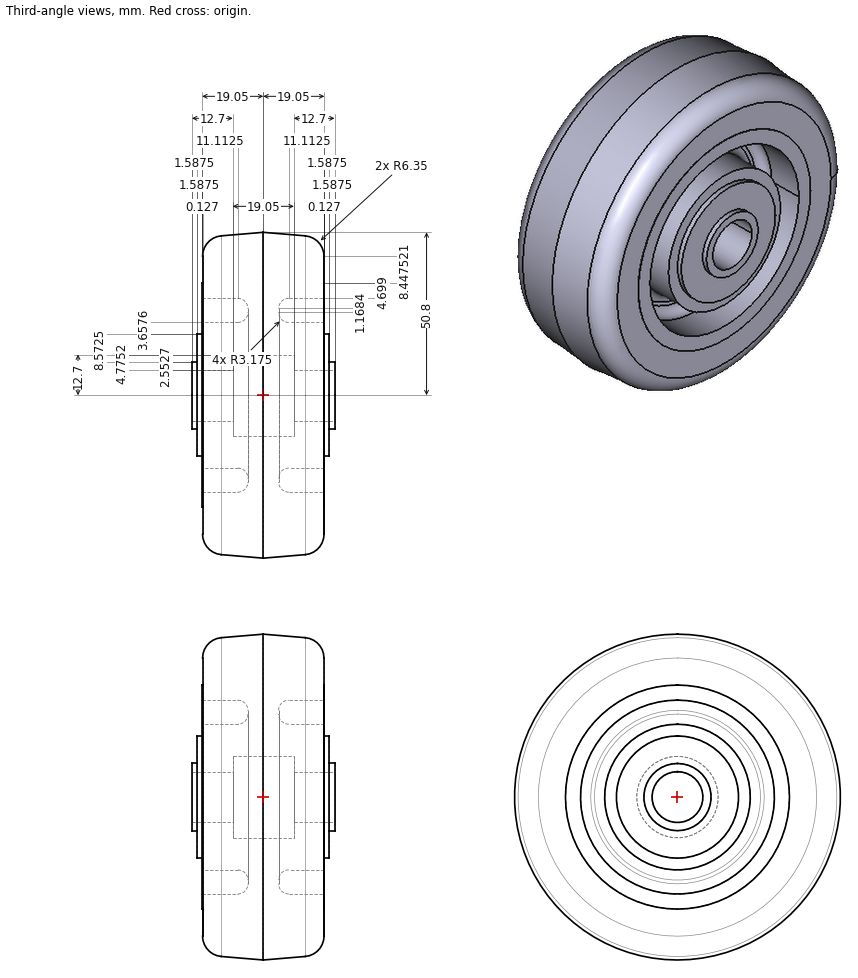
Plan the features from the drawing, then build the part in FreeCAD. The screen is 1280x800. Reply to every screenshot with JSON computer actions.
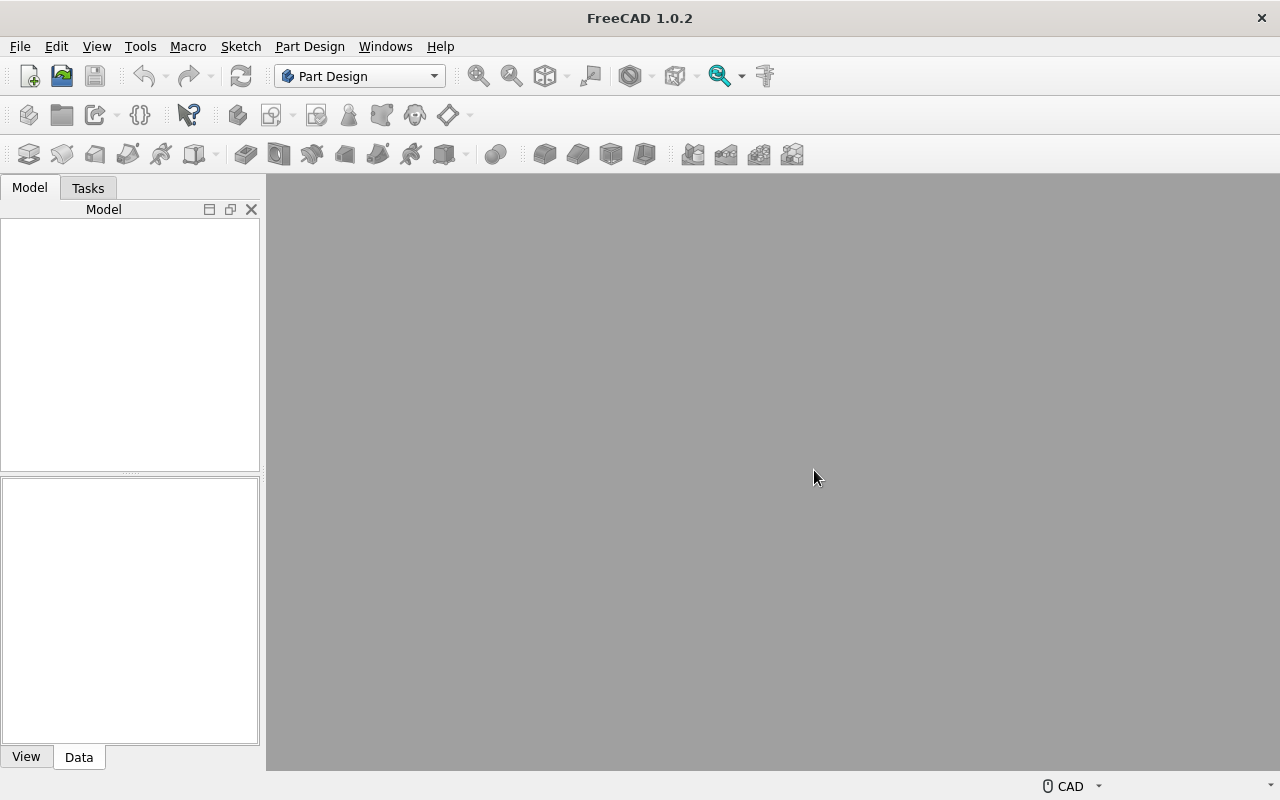
{"action": "left_click", "coordinate": [29, 76]}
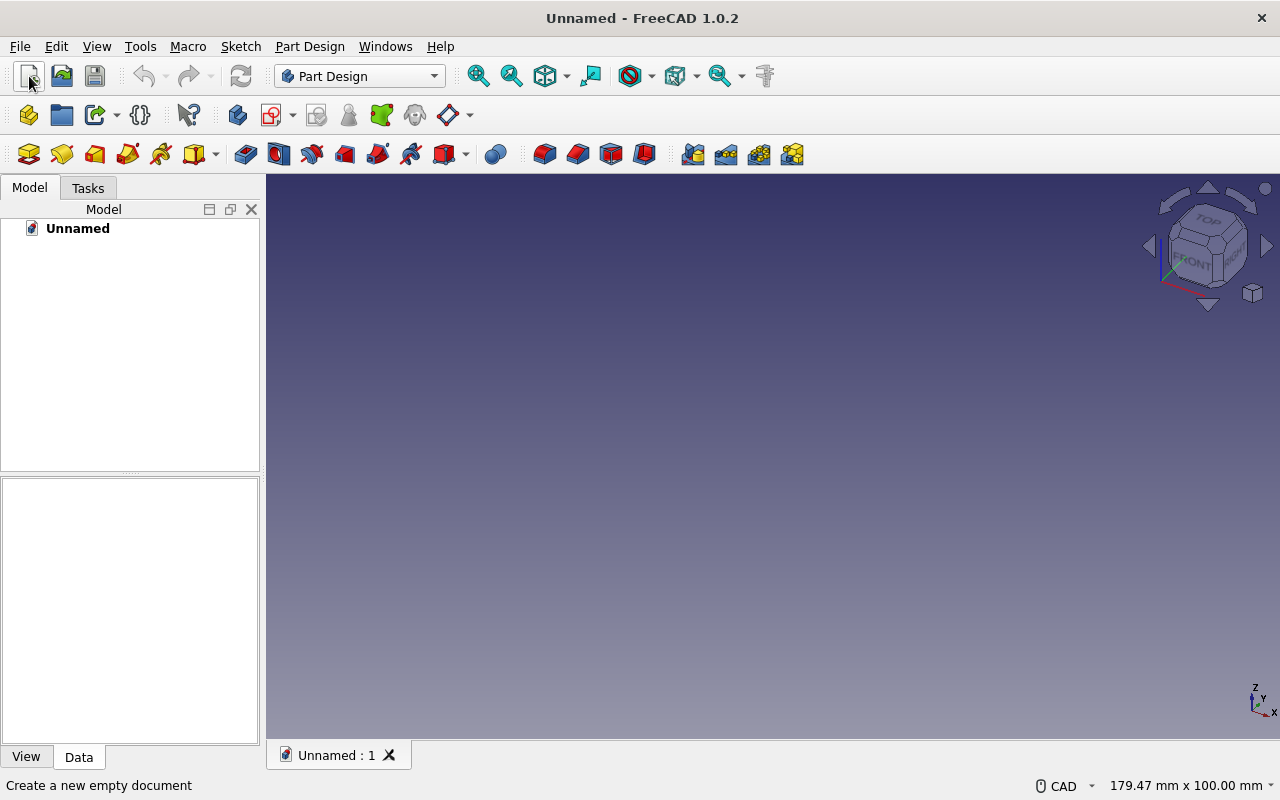
{"action": "left_click", "coordinate": [270, 116]}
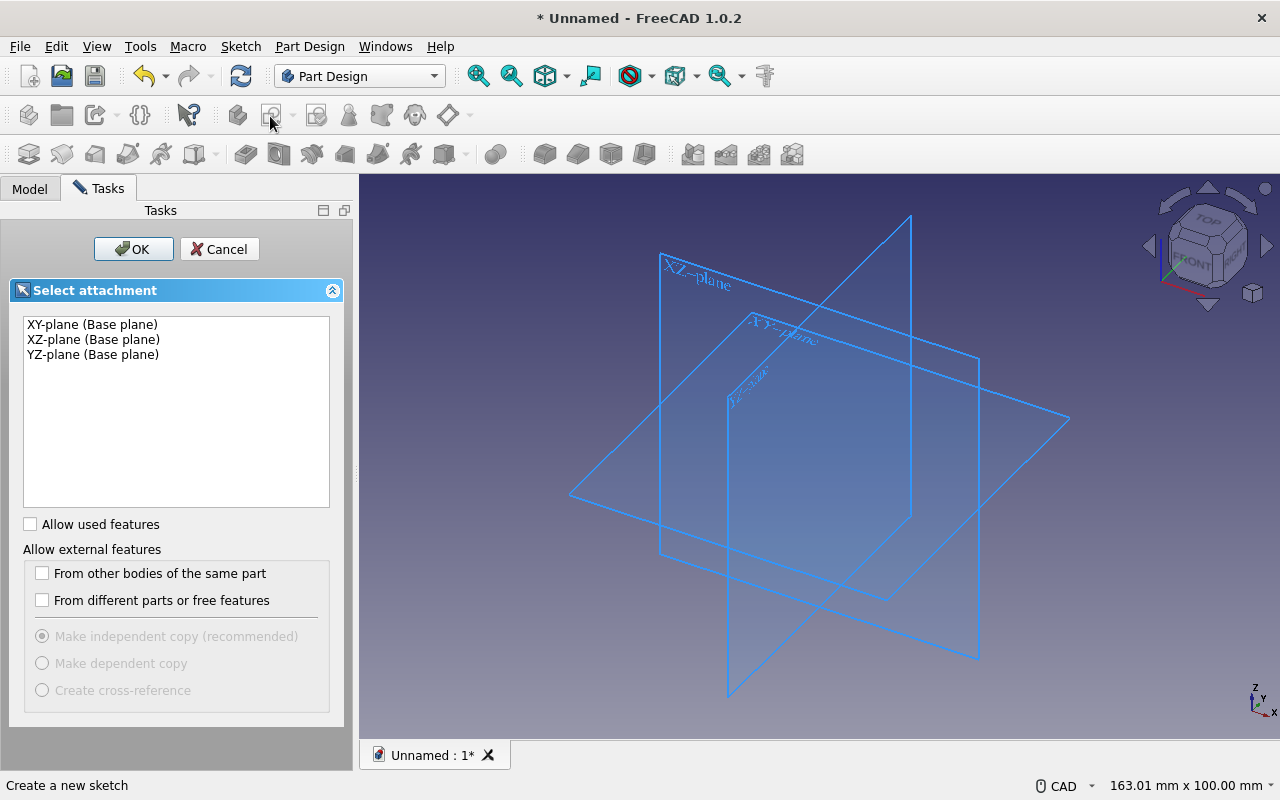
{"action": "left_click", "coordinate": [84, 324]}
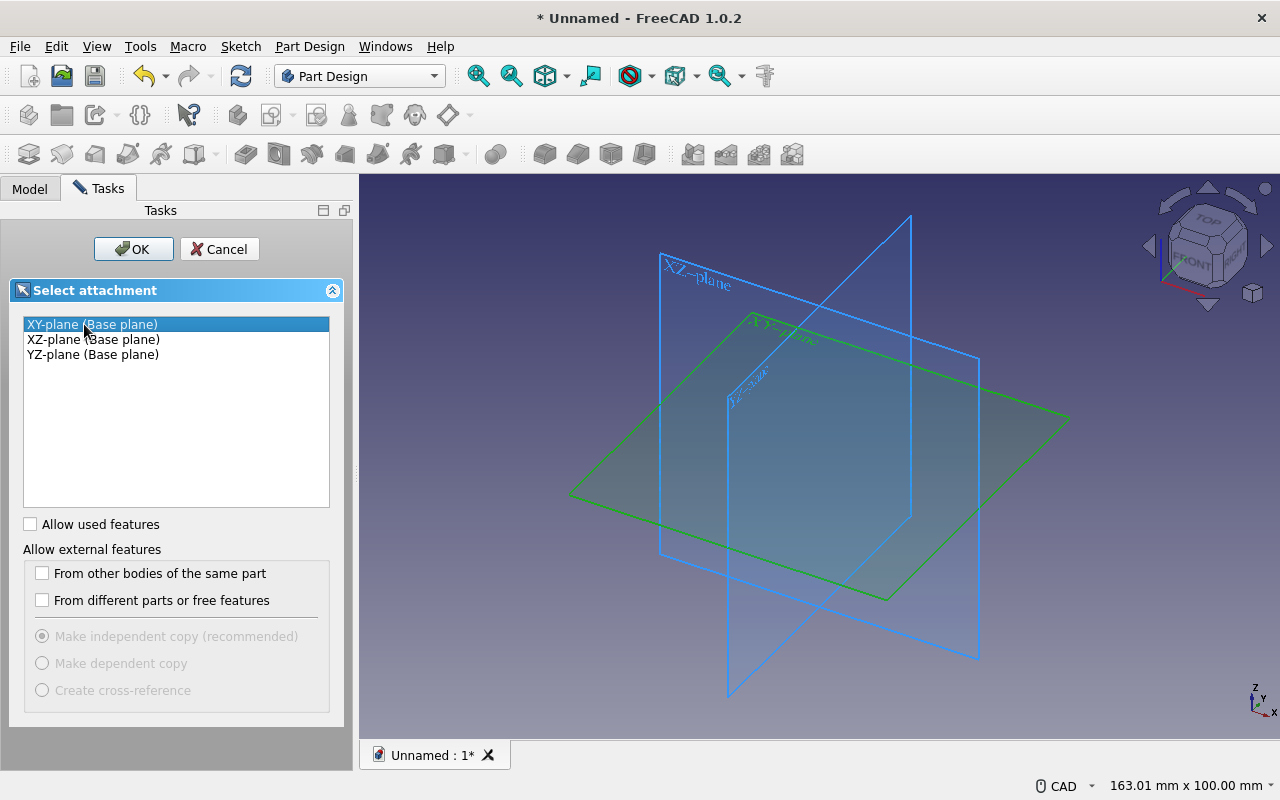
{"action": "left_click", "coordinate": [134, 249]}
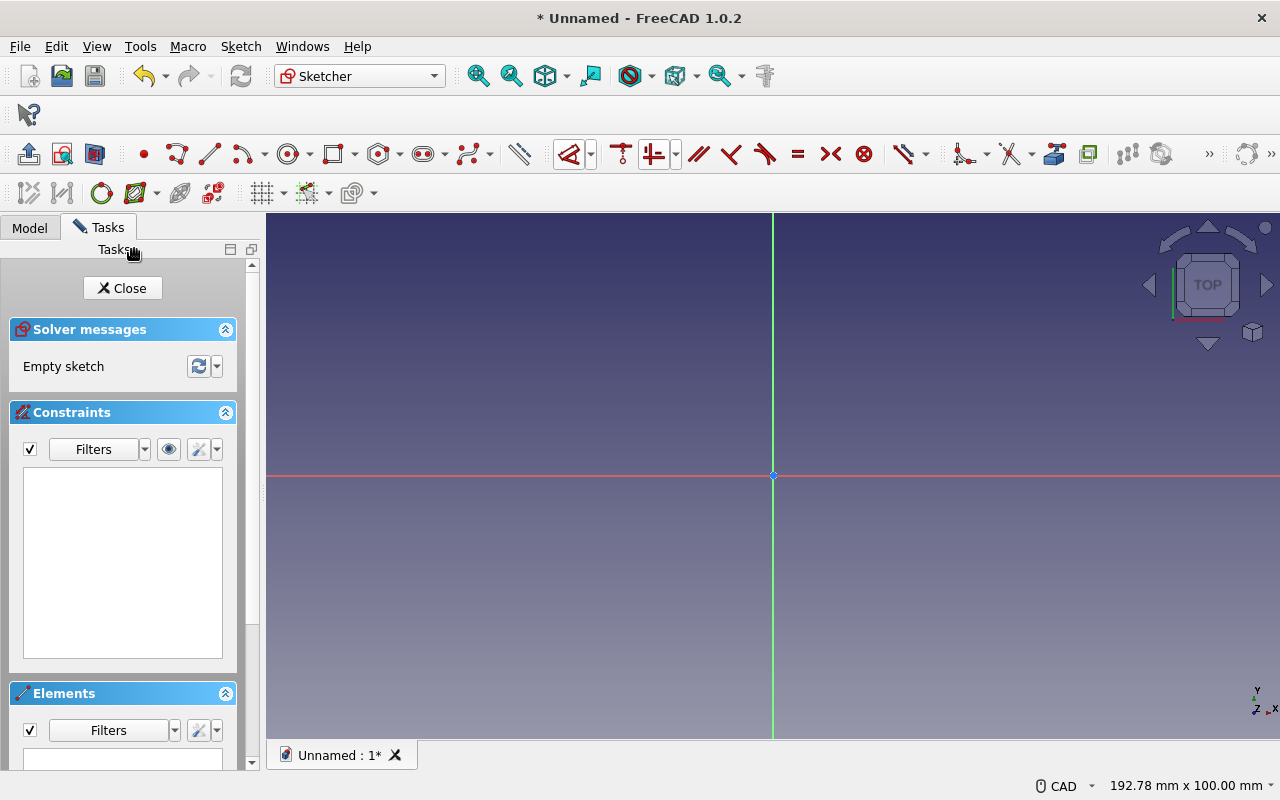
{"action": "scroll", "coordinate": [395, 711], "scroll_direction": "down", "scroll_amount": 1}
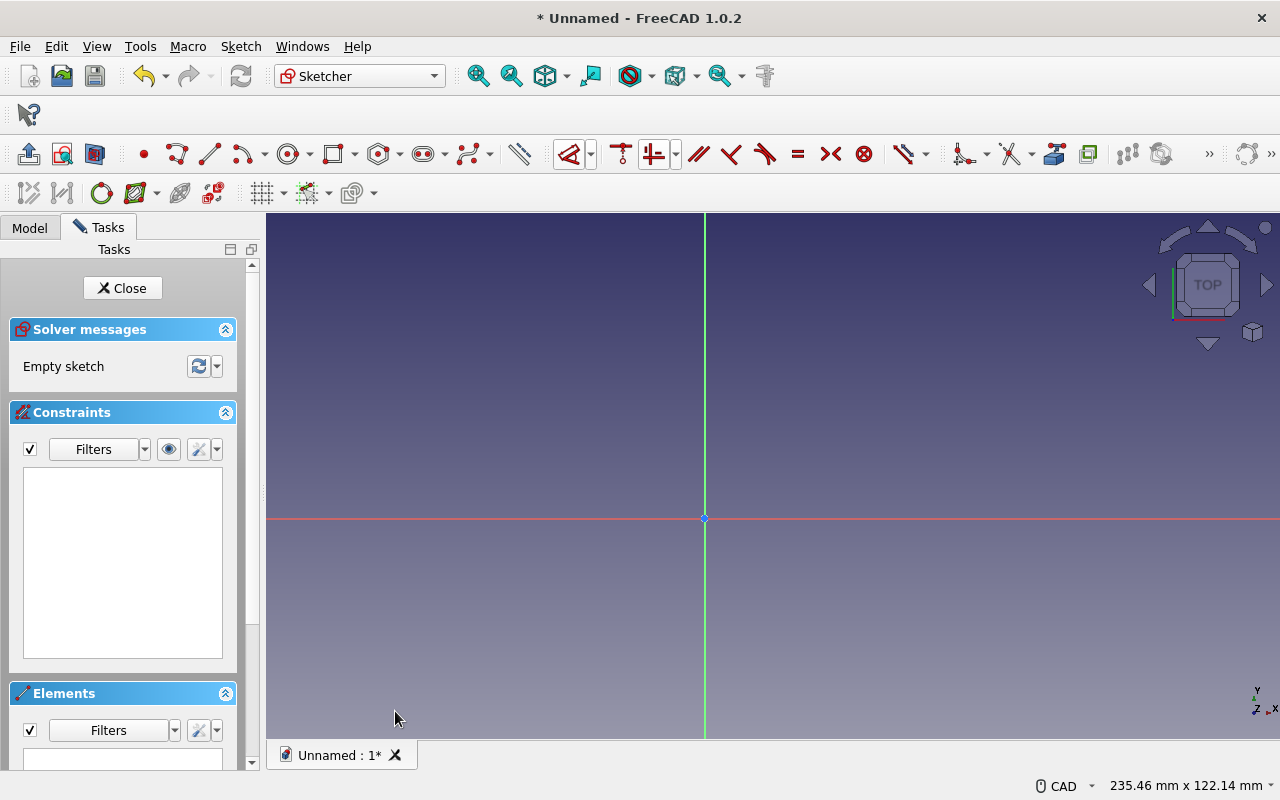
{"action": "scroll", "coordinate": [705, 274], "scroll_direction": "up", "scroll_amount": 2}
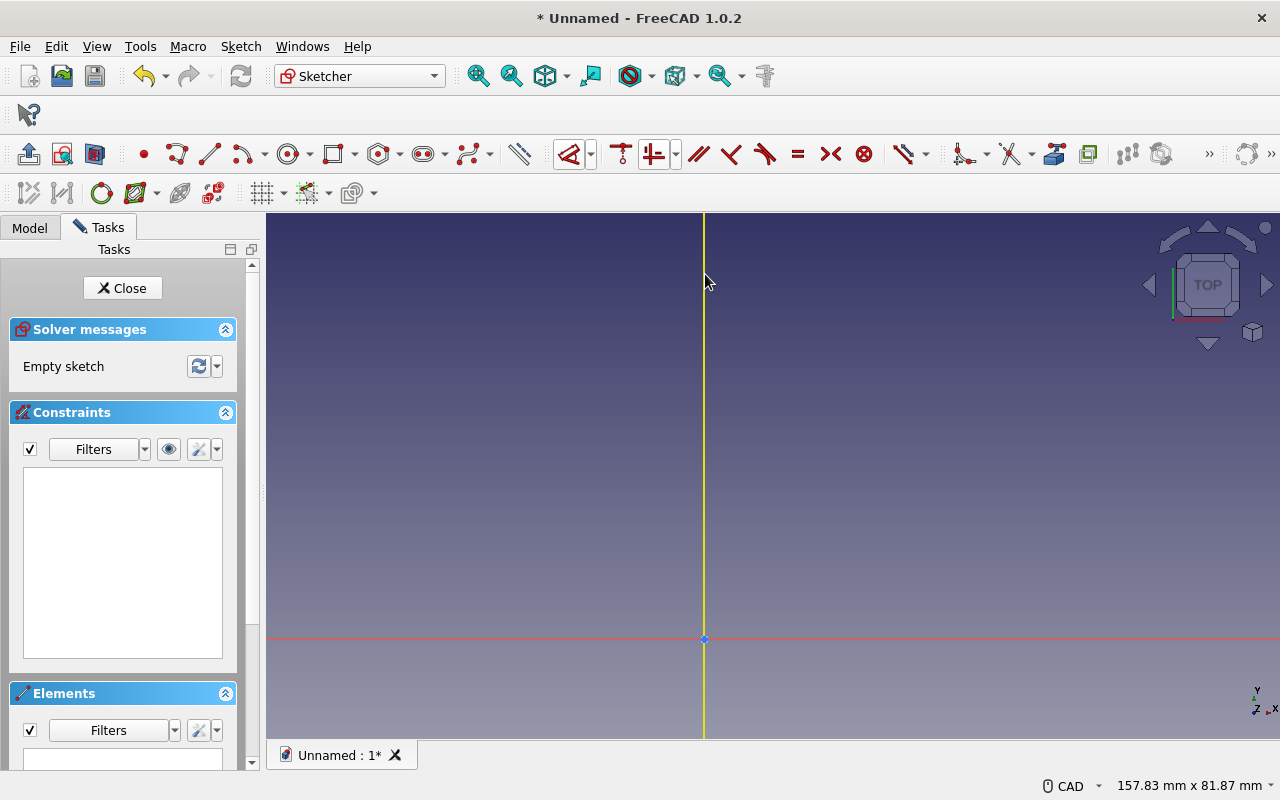
{"action": "left_click", "coordinate": [210, 154]}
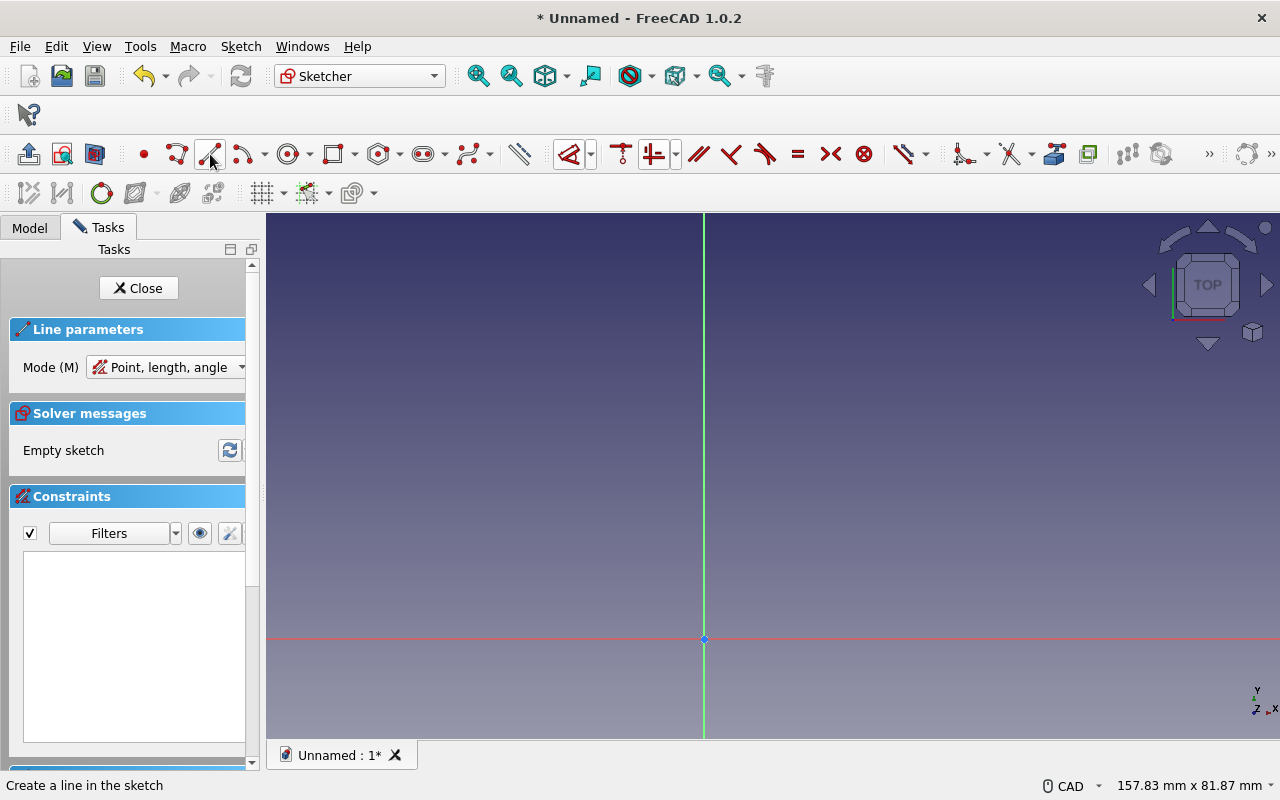
{"action": "left_click", "coordinate": [735, 473]}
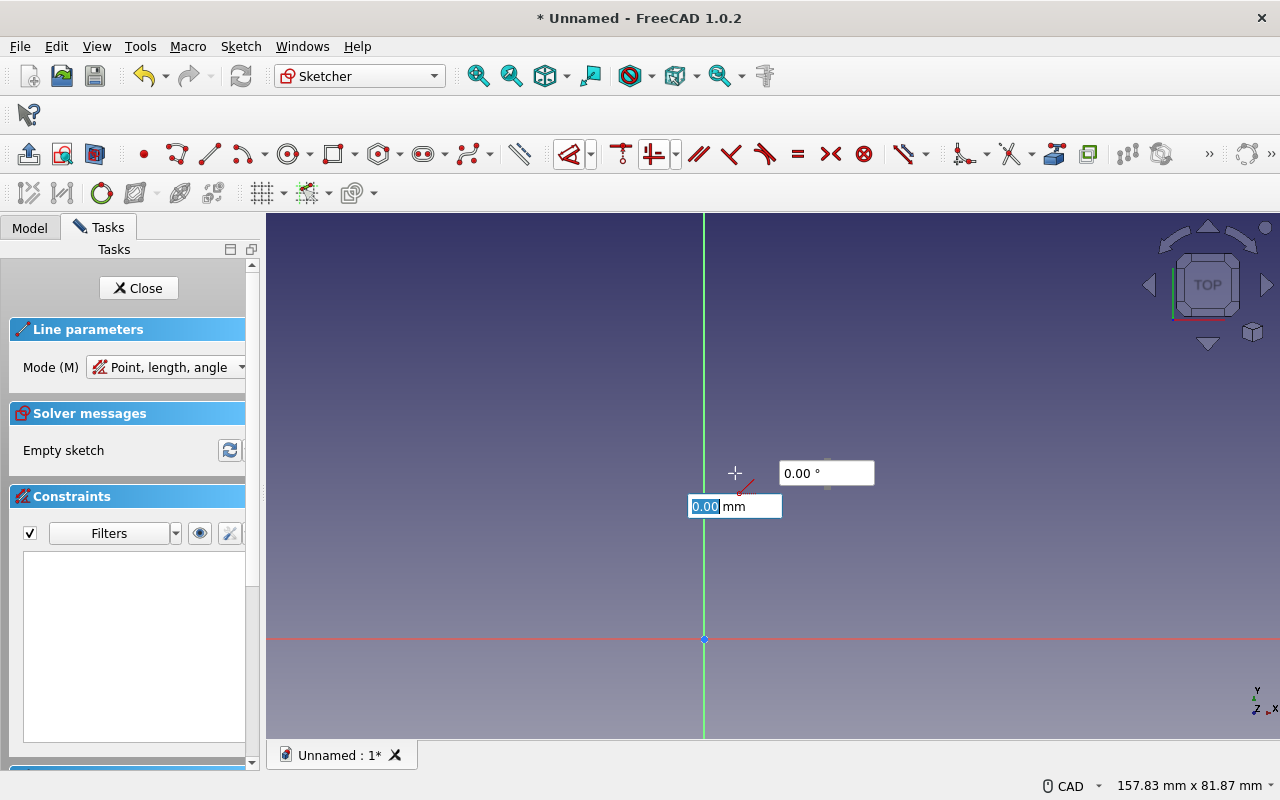
{"action": "scroll", "coordinate": [735, 465], "scroll_direction": "up", "scroll_amount": 4}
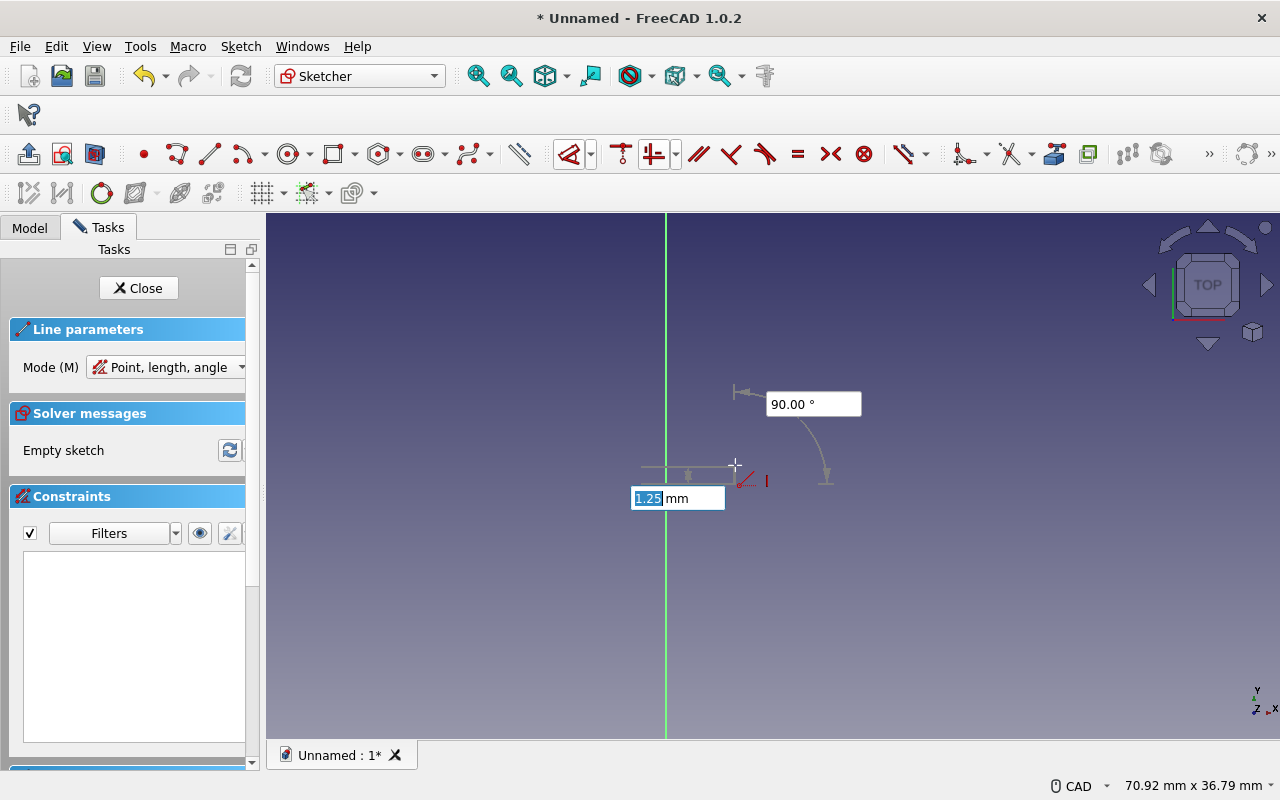
{"action": "left_click", "coordinate": [734, 465]}